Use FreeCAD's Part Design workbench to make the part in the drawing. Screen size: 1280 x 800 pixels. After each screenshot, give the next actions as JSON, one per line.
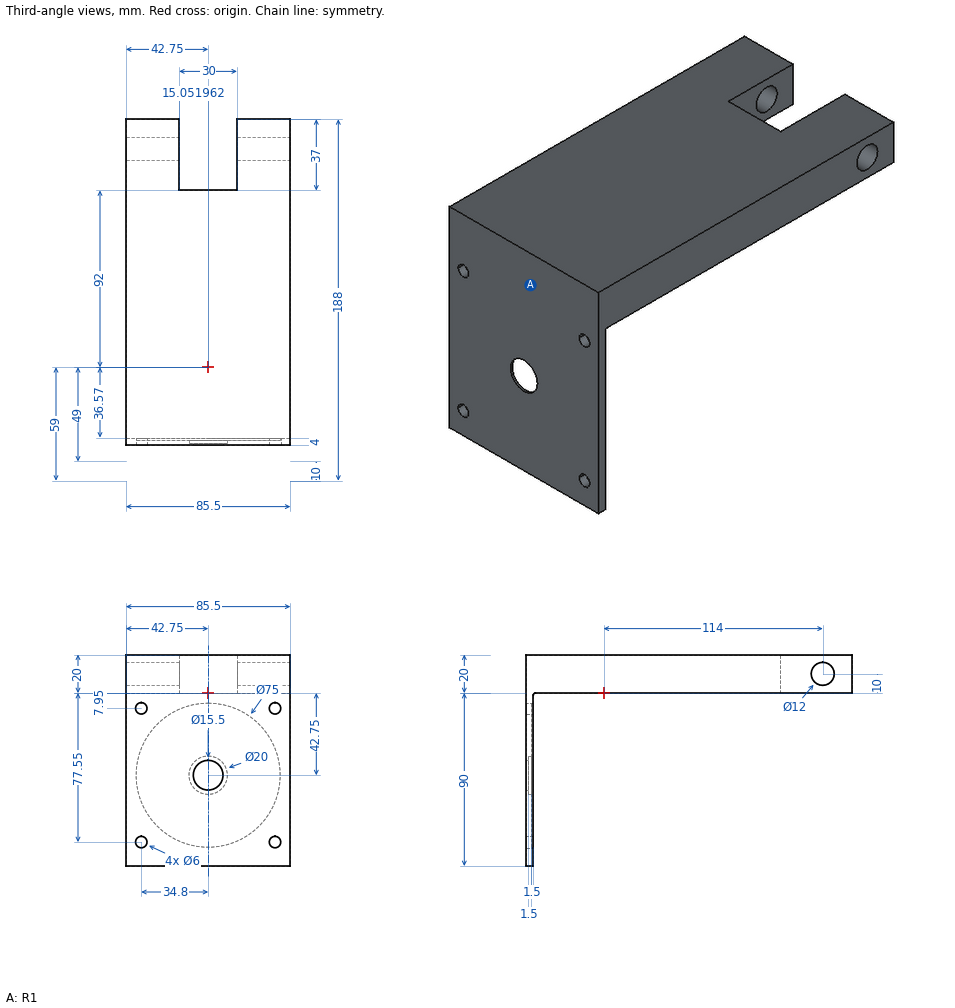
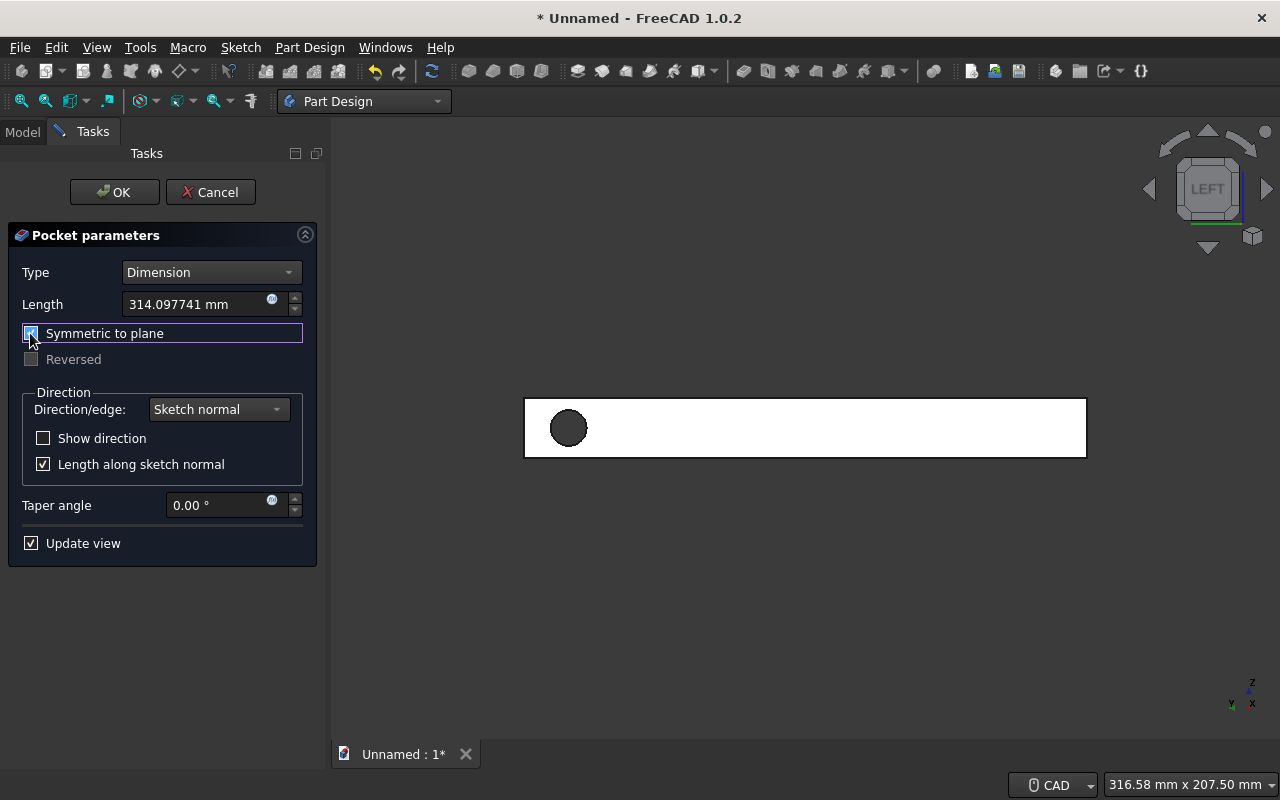
{"action": "left_click", "coordinate": [115, 192]}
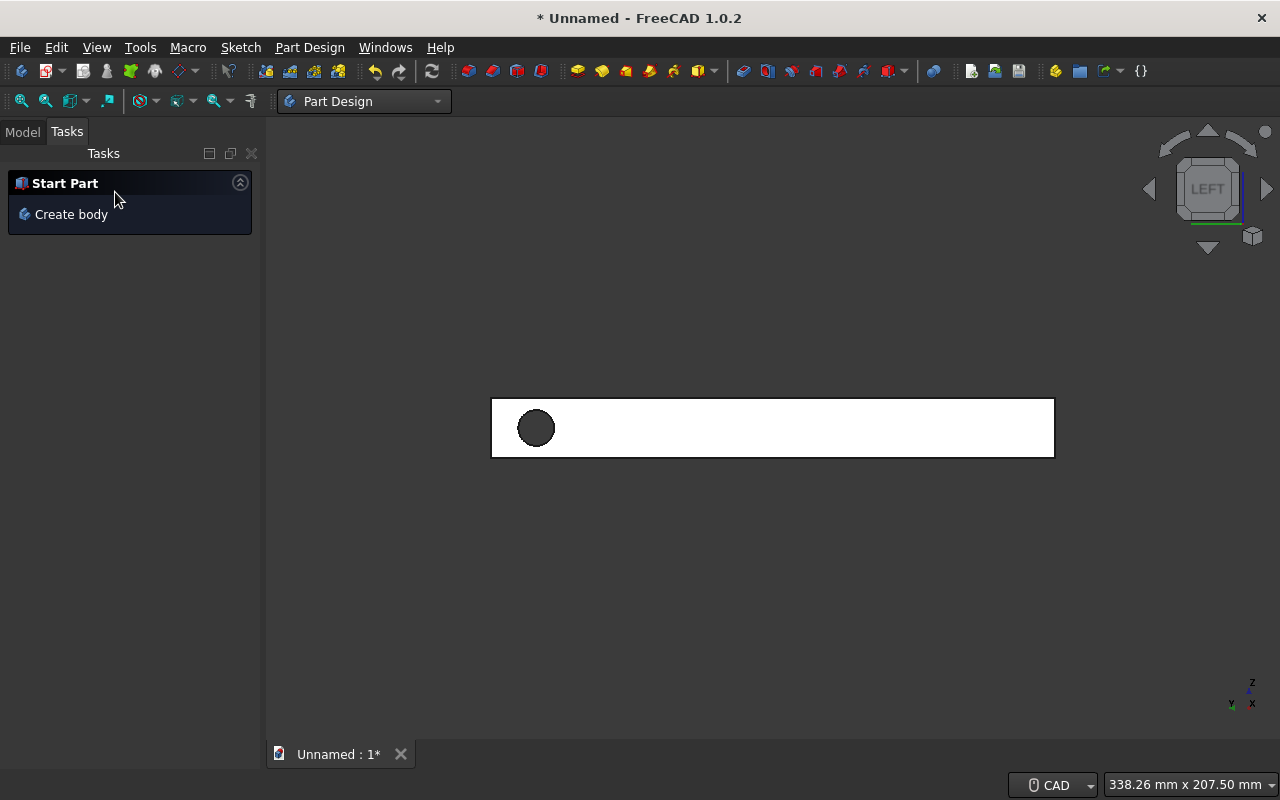
{"action": "key", "text": "0"}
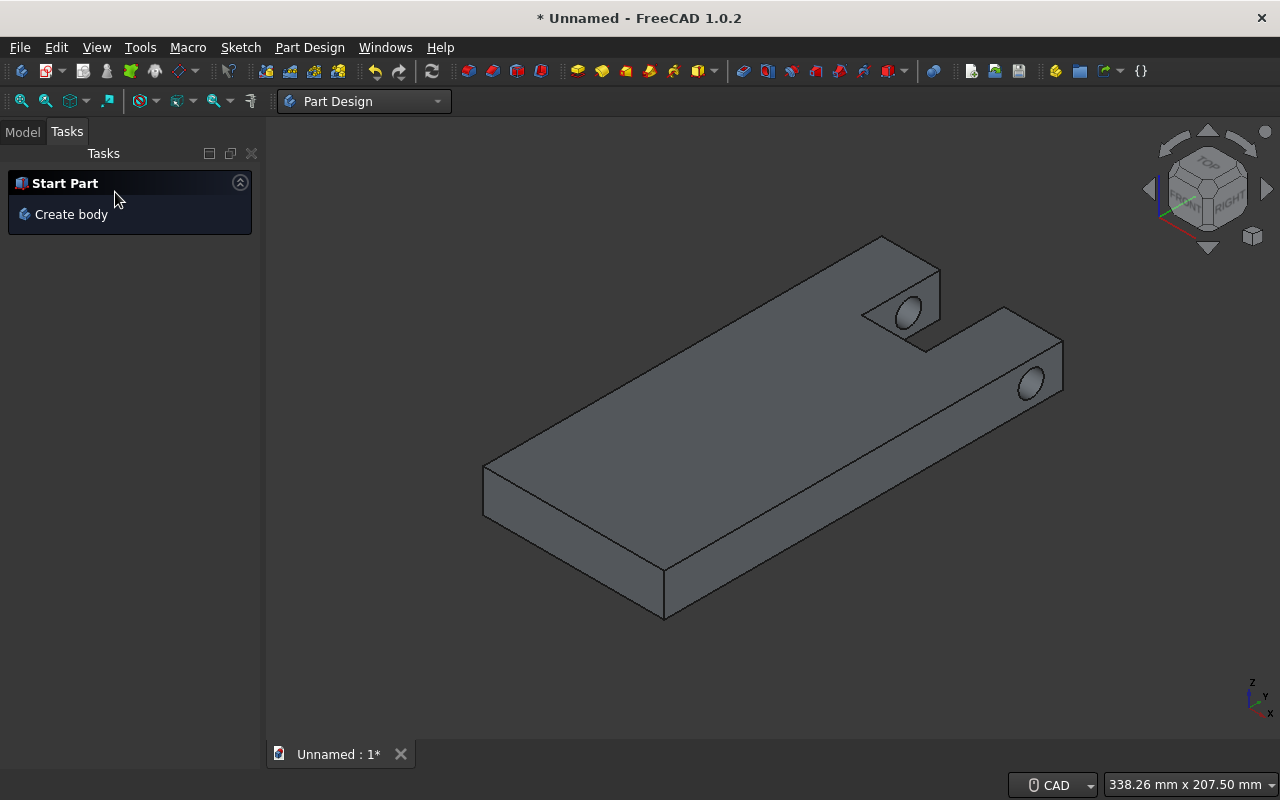
{"action": "left_click", "coordinate": [773, 403]}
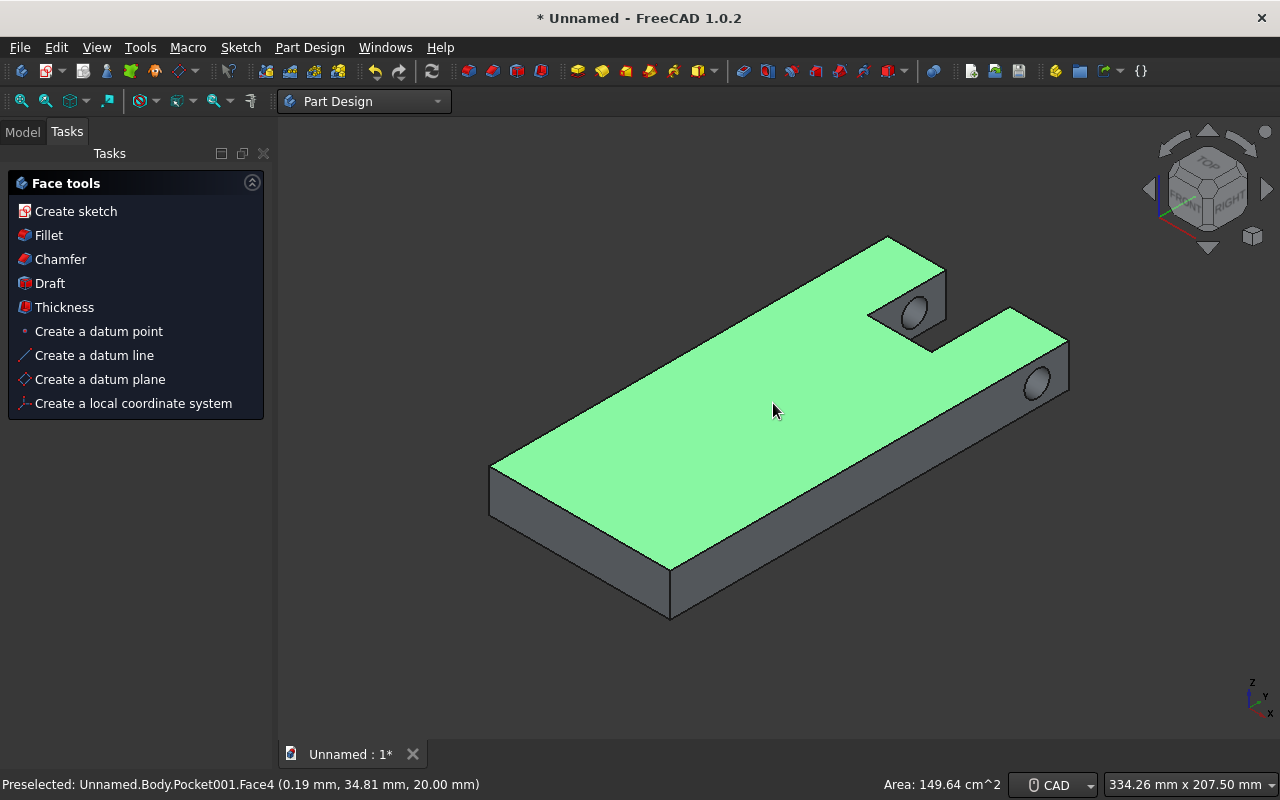
{"action": "left_click", "coordinate": [46, 72]}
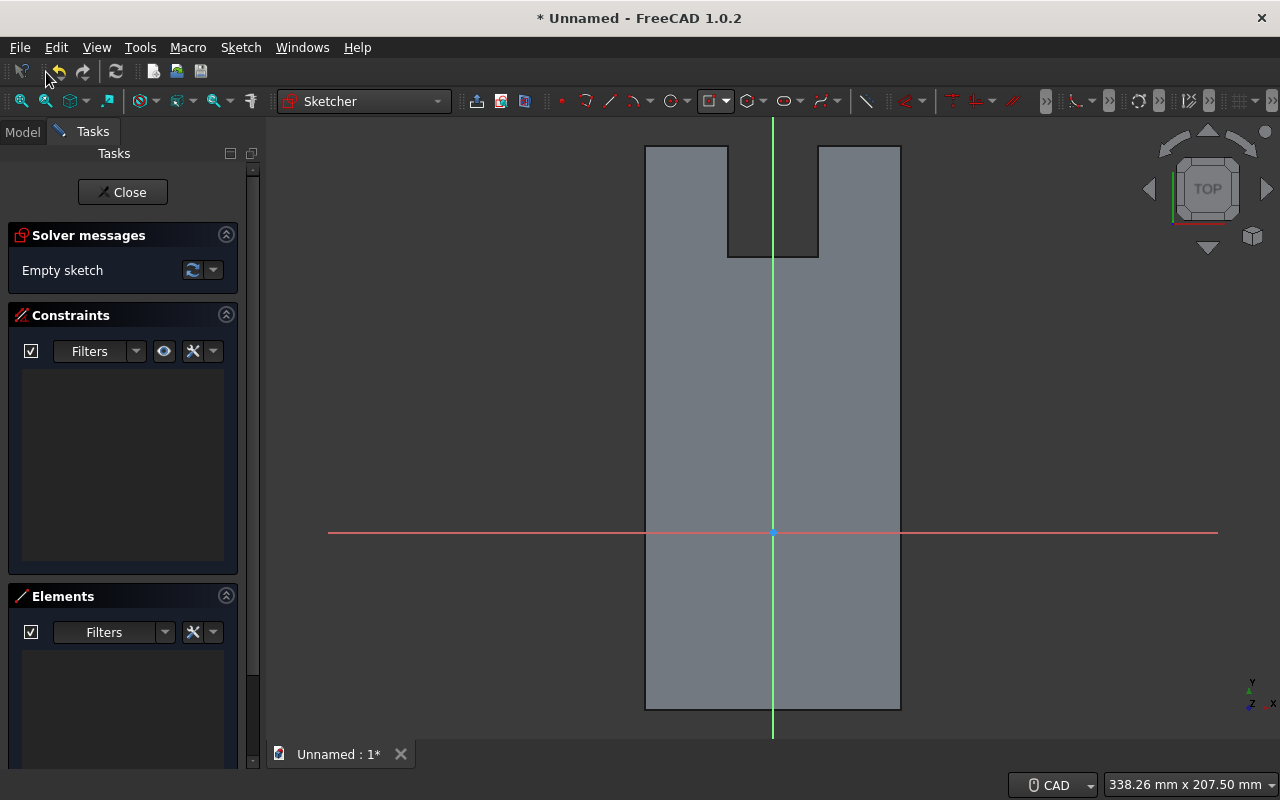
{"action": "scroll", "coordinate": [704, 428], "scroll_direction": "down", "scroll_amount": 5}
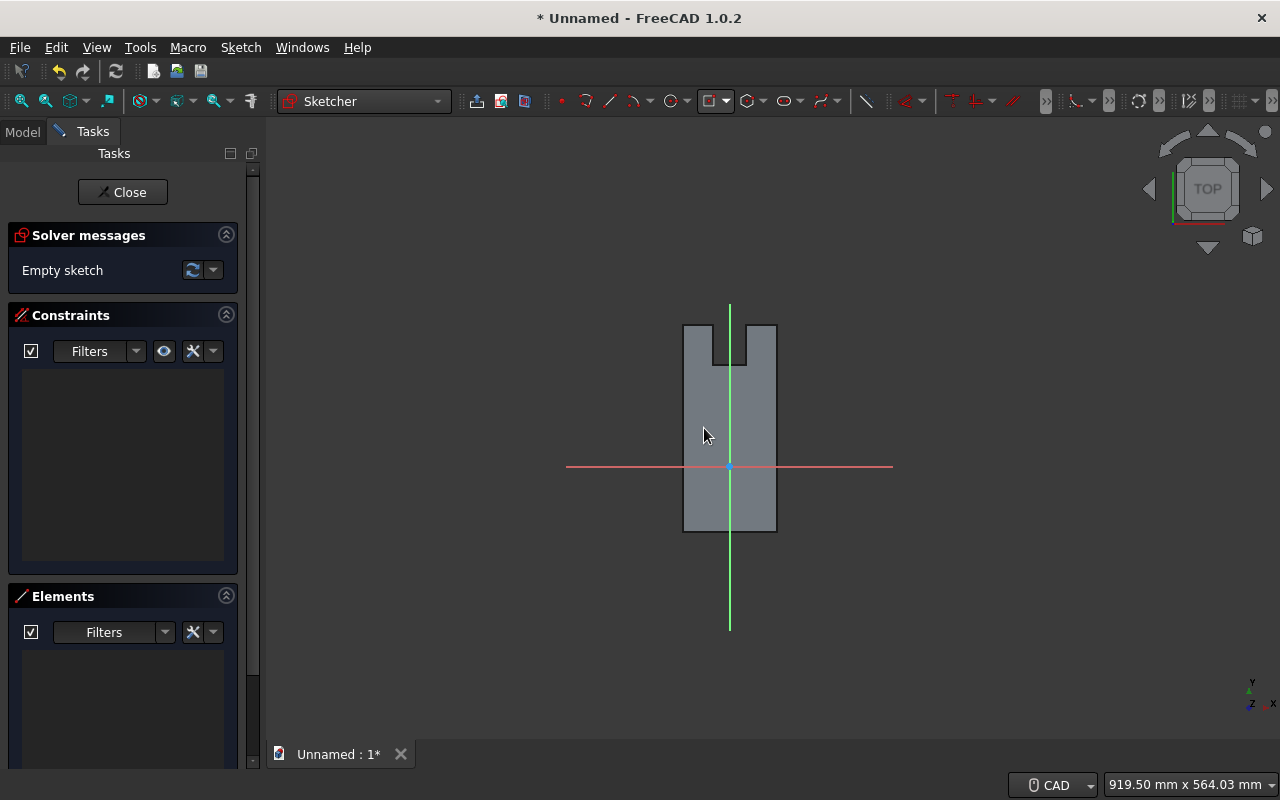
{"action": "scroll", "coordinate": [735, 514], "scroll_direction": "up", "scroll_amount": 9}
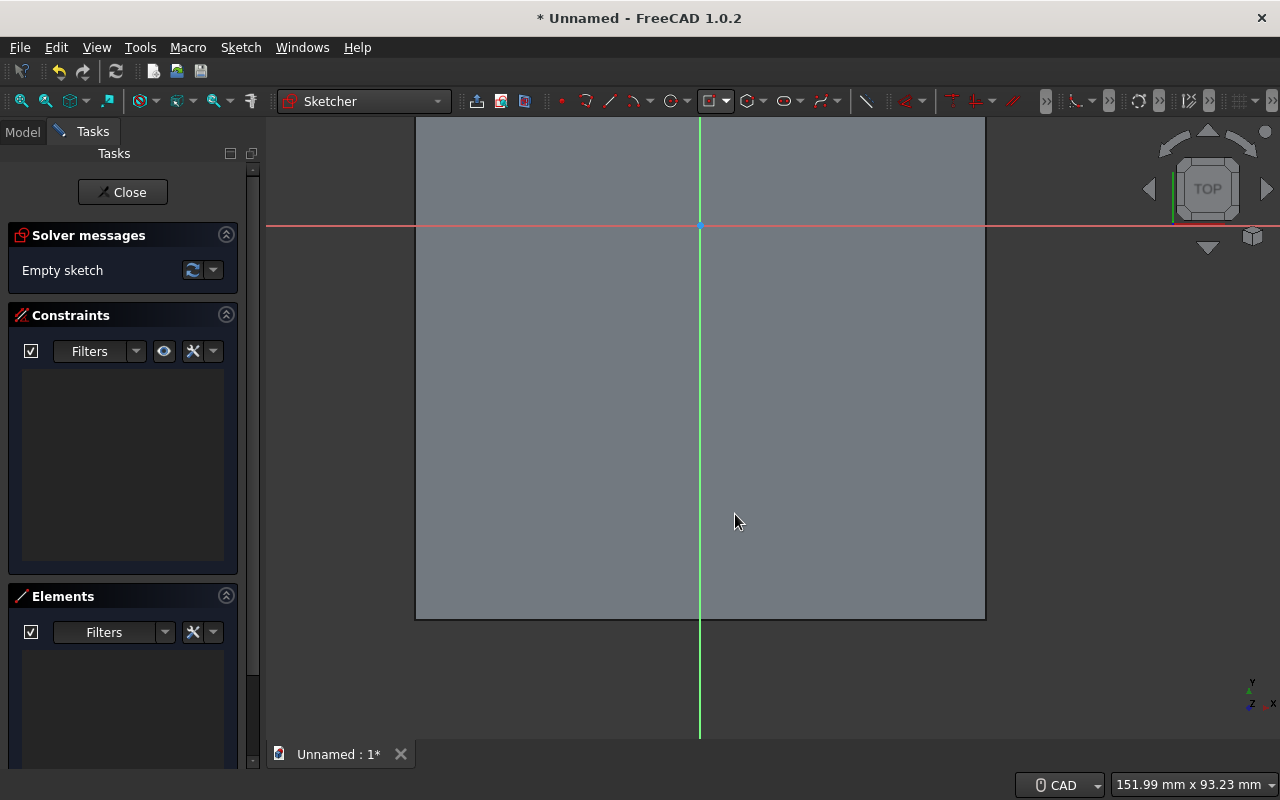
{"action": "key", "text": "g r"}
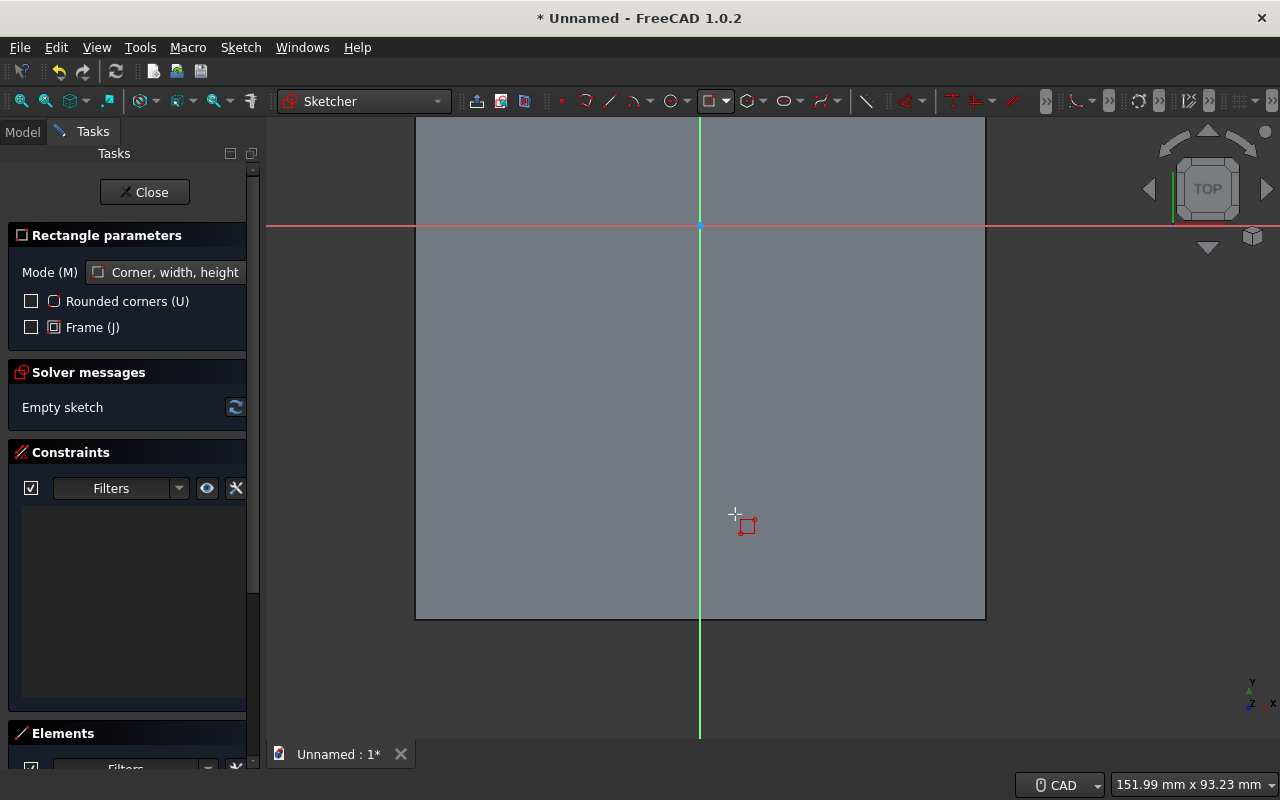
{"action": "left_click", "coordinate": [415, 553]}
{"action": "mouse_move", "coordinate": [986, 620]}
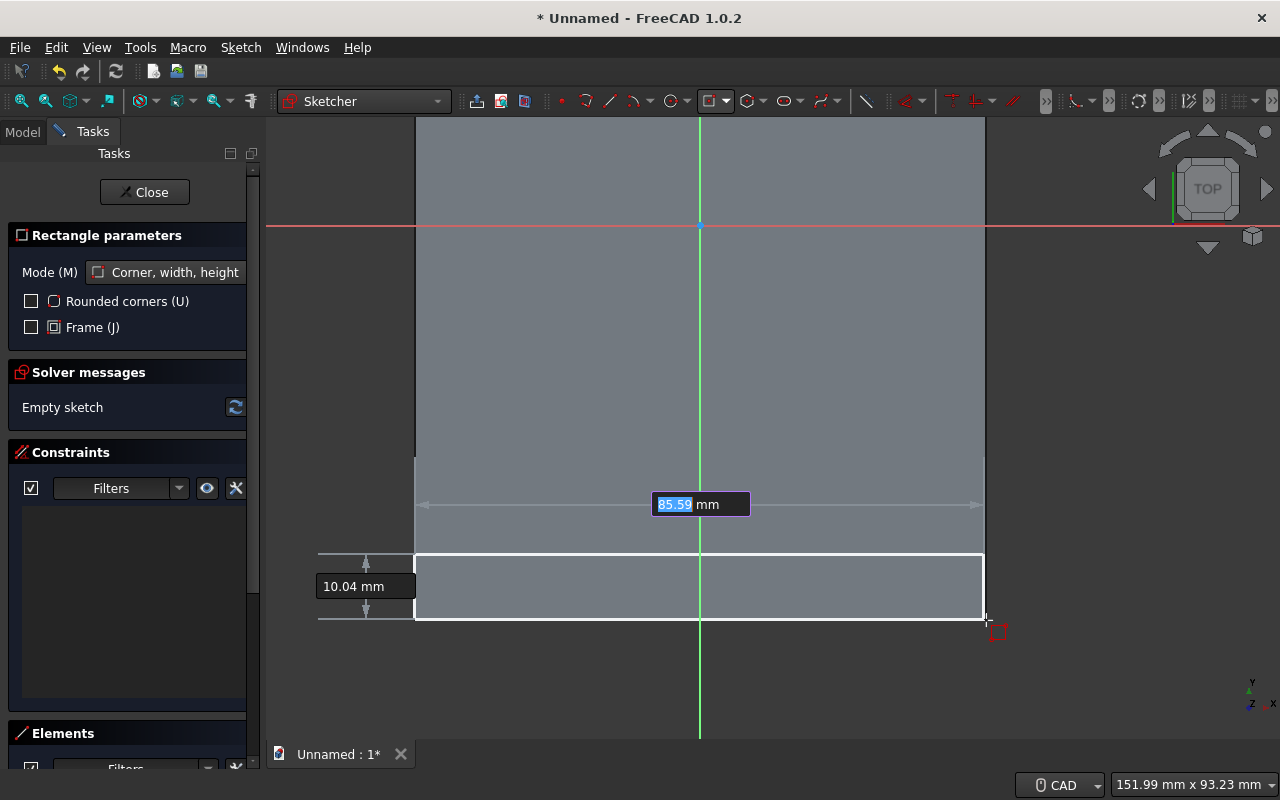
{"action": "type", "text": "85.5"}
{"action": "key", "text": "Tab"}
{"action": "type", "text": "10"}
{"action": "key", "text": "Return"}
{"action": "key", "text": "Escape"}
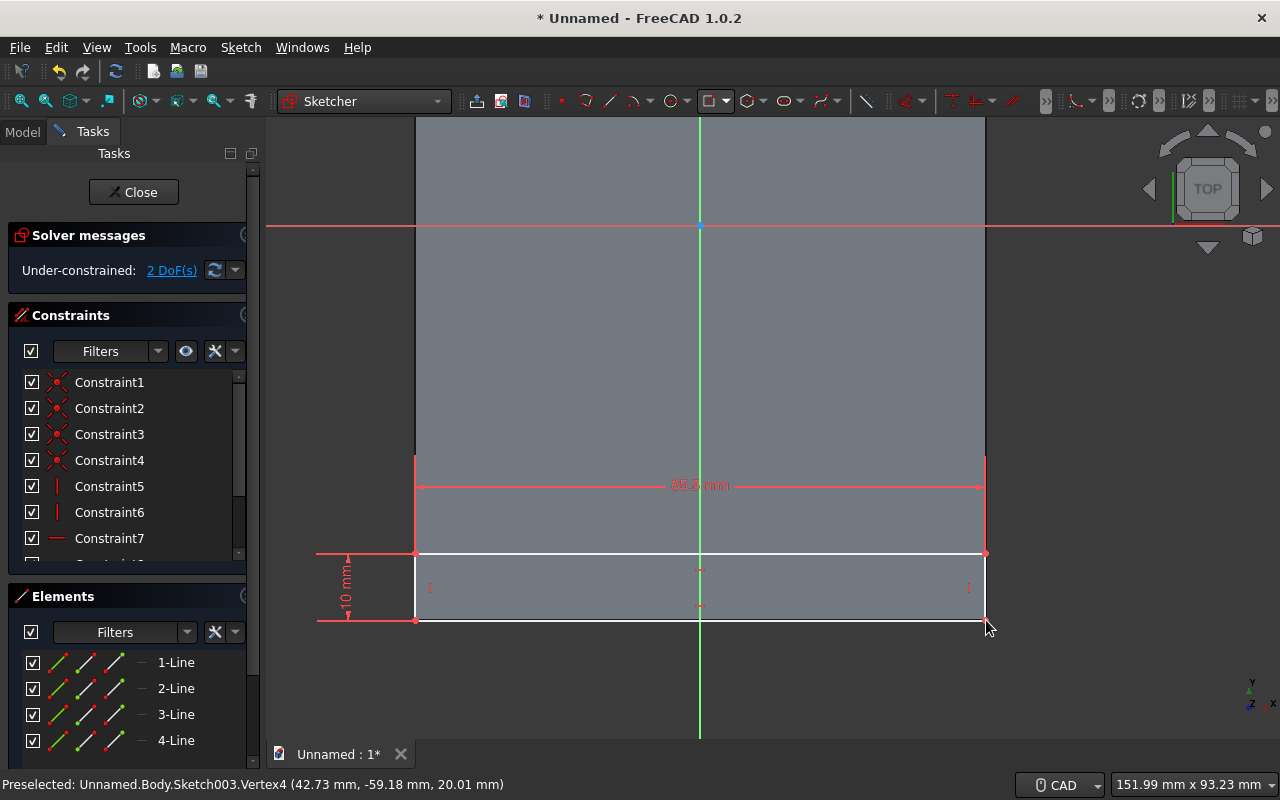
{"action": "left_click", "coordinate": [906, 102]}